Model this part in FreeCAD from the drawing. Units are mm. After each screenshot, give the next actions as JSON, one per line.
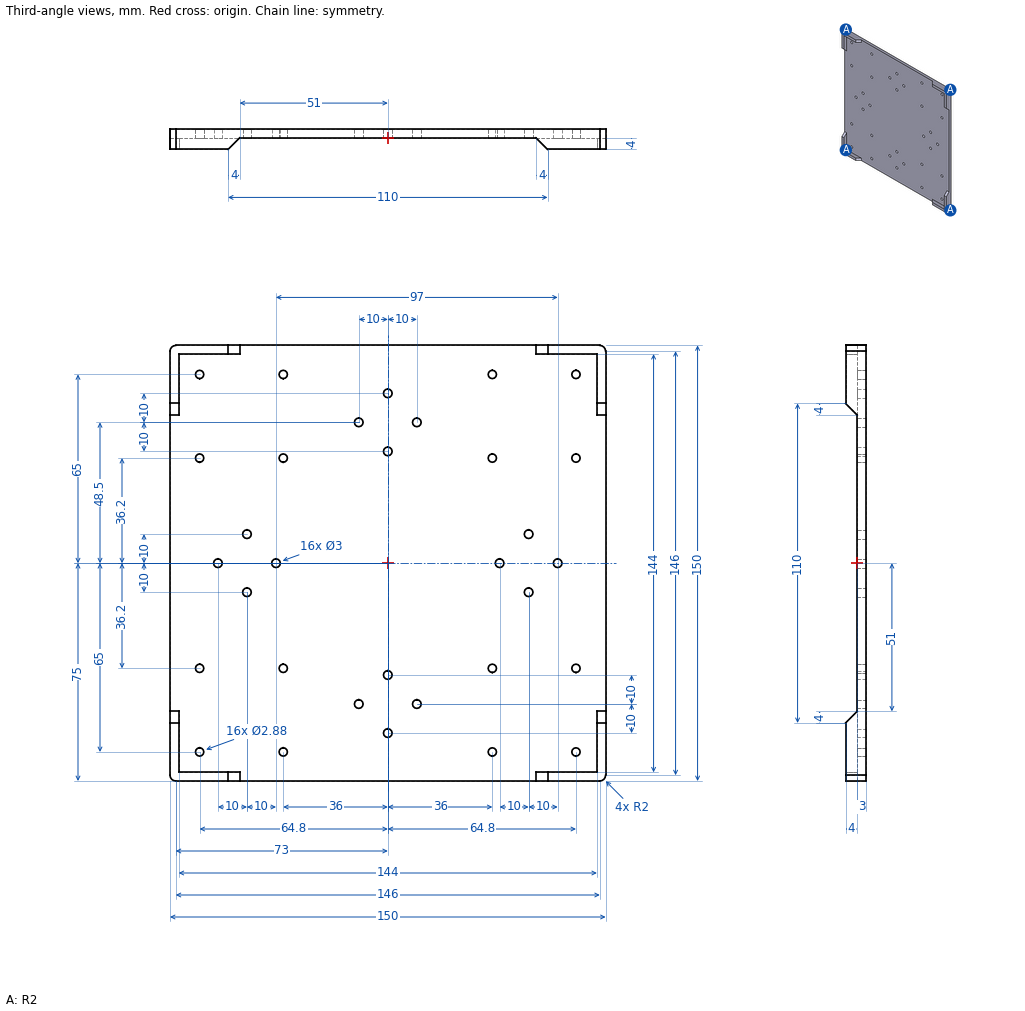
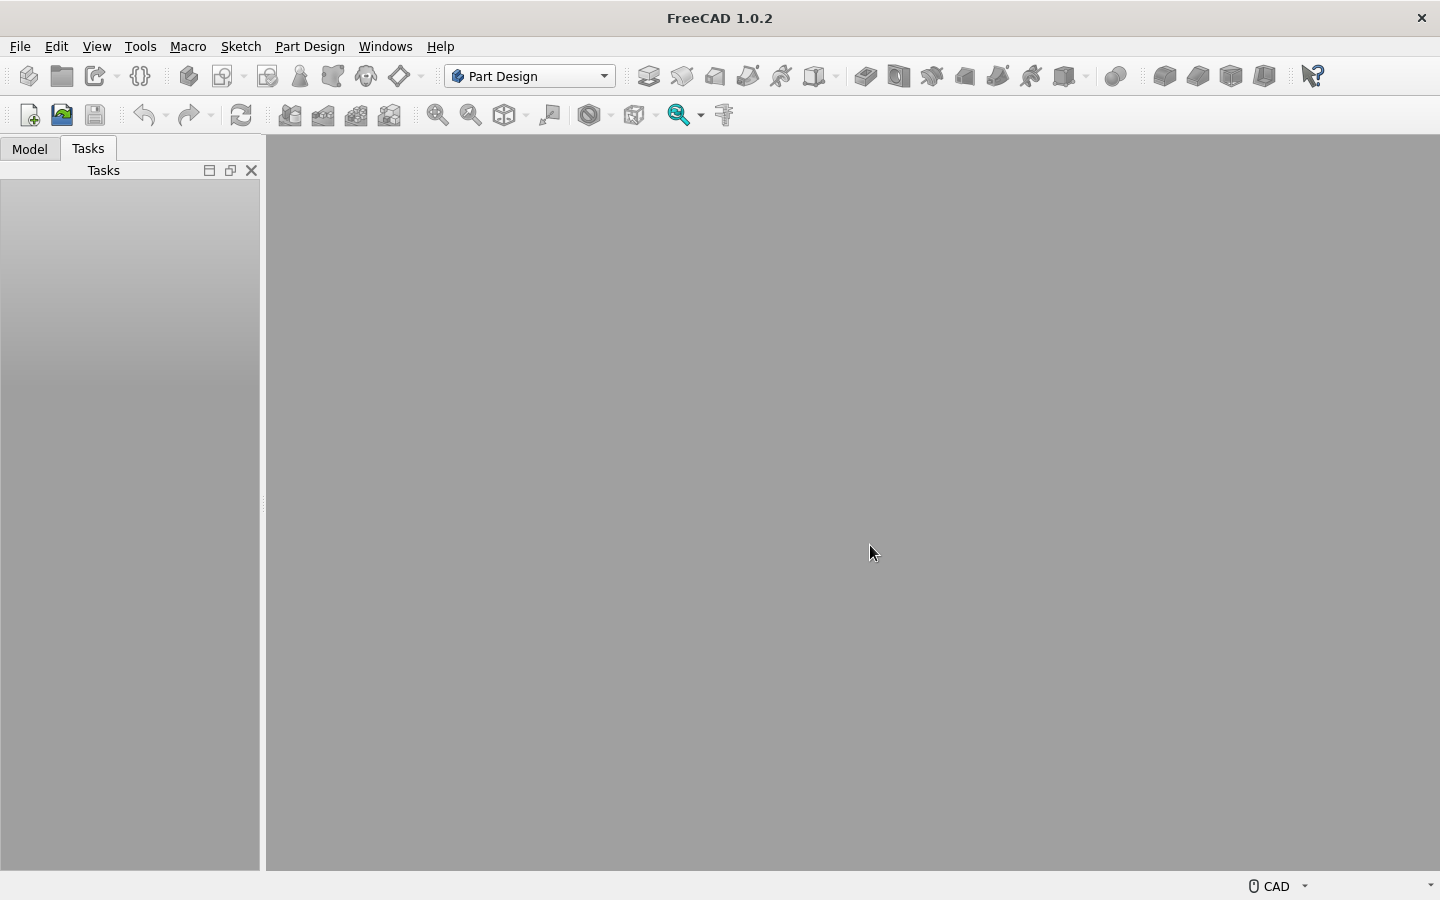
{"action": "left_click", "coordinate": [29, 116]}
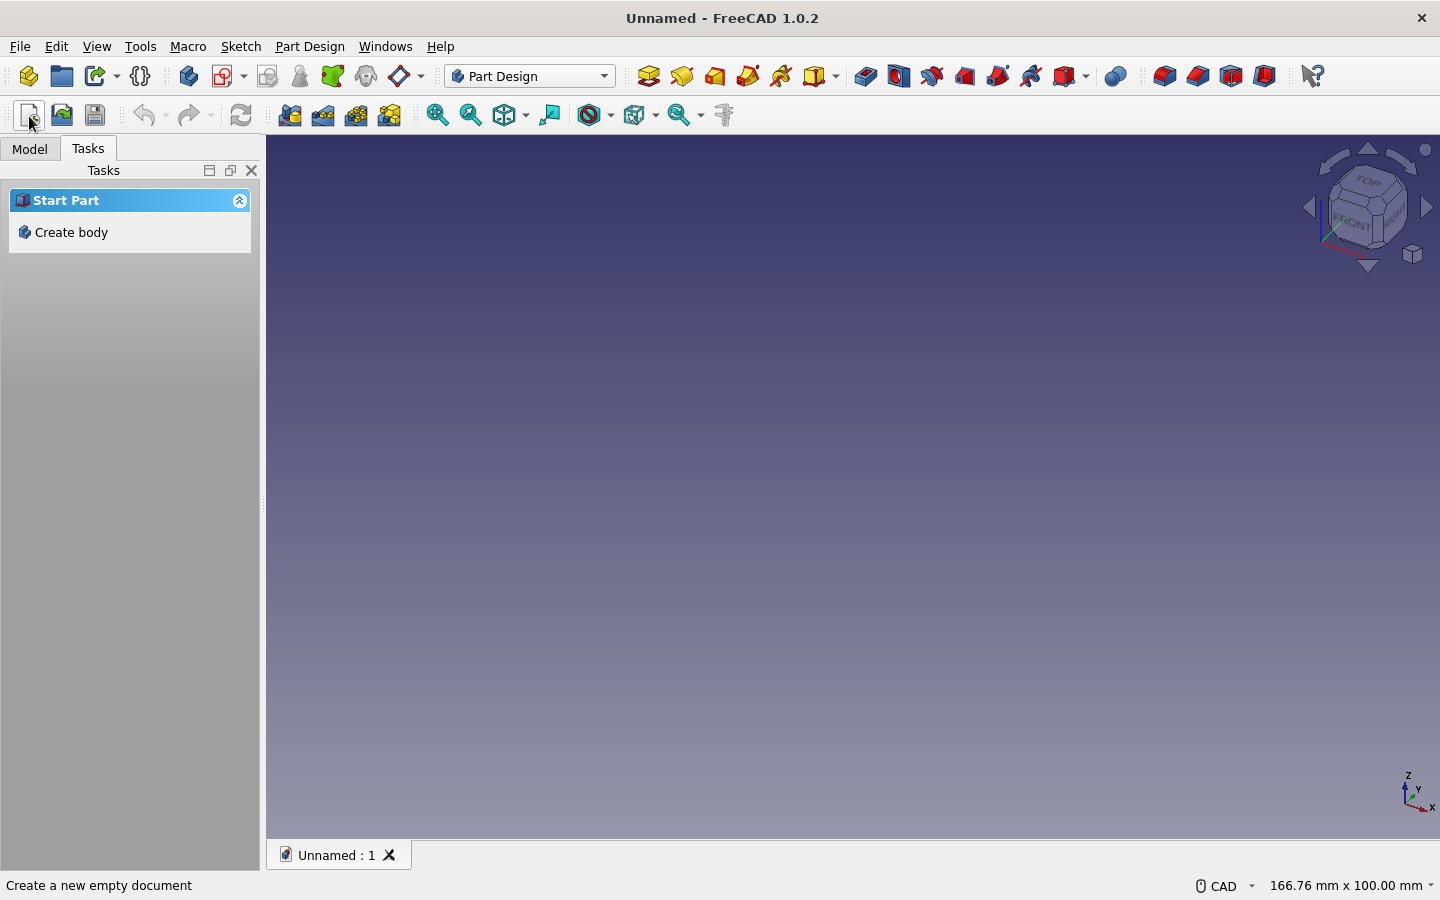
{"action": "left_click", "coordinate": [222, 76]}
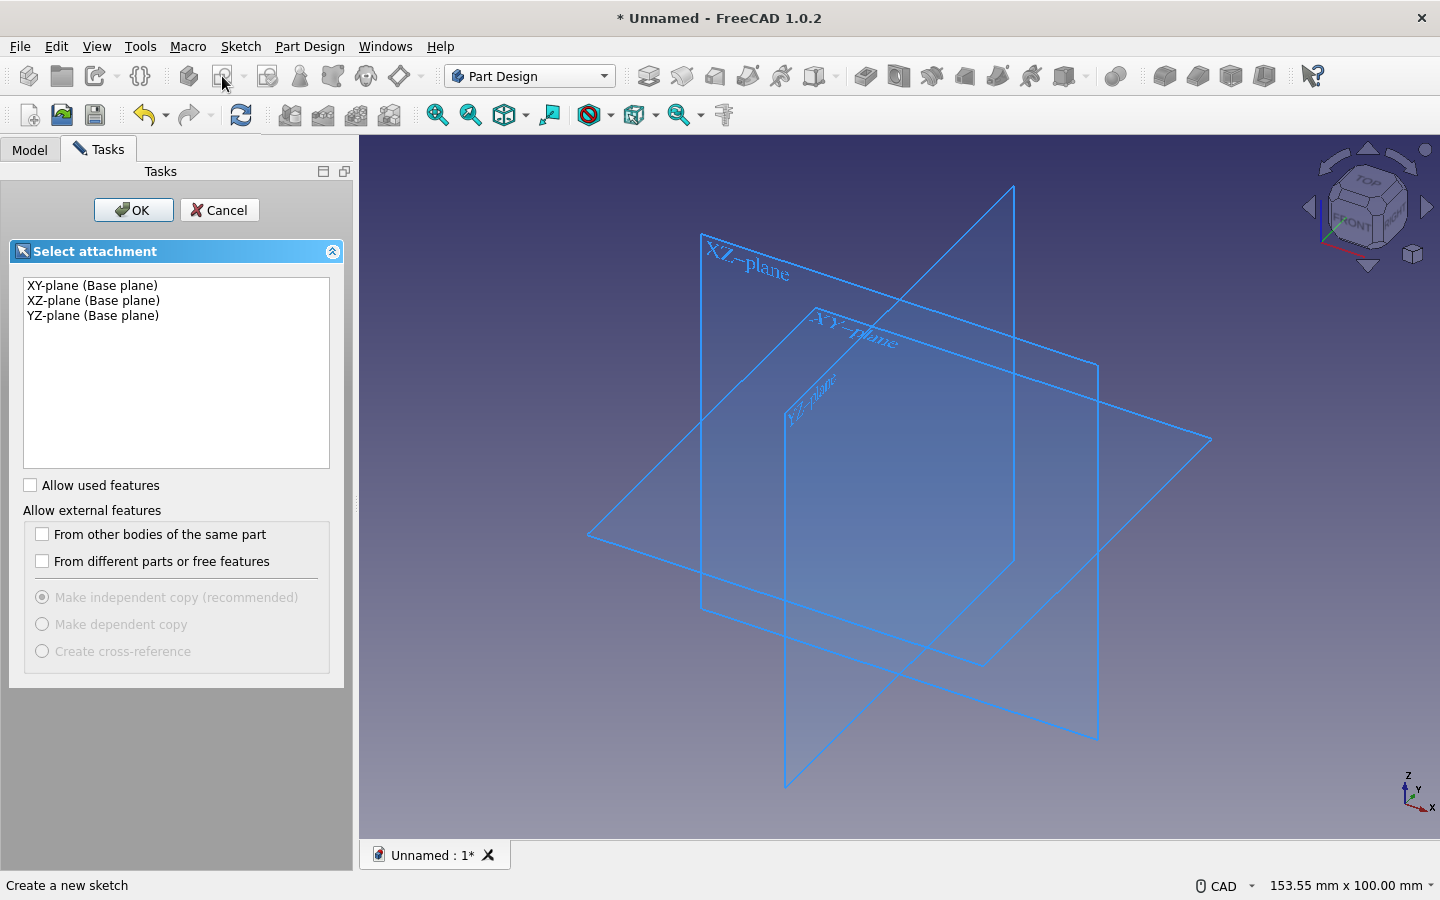
{"action": "left_click", "coordinate": [84, 300]}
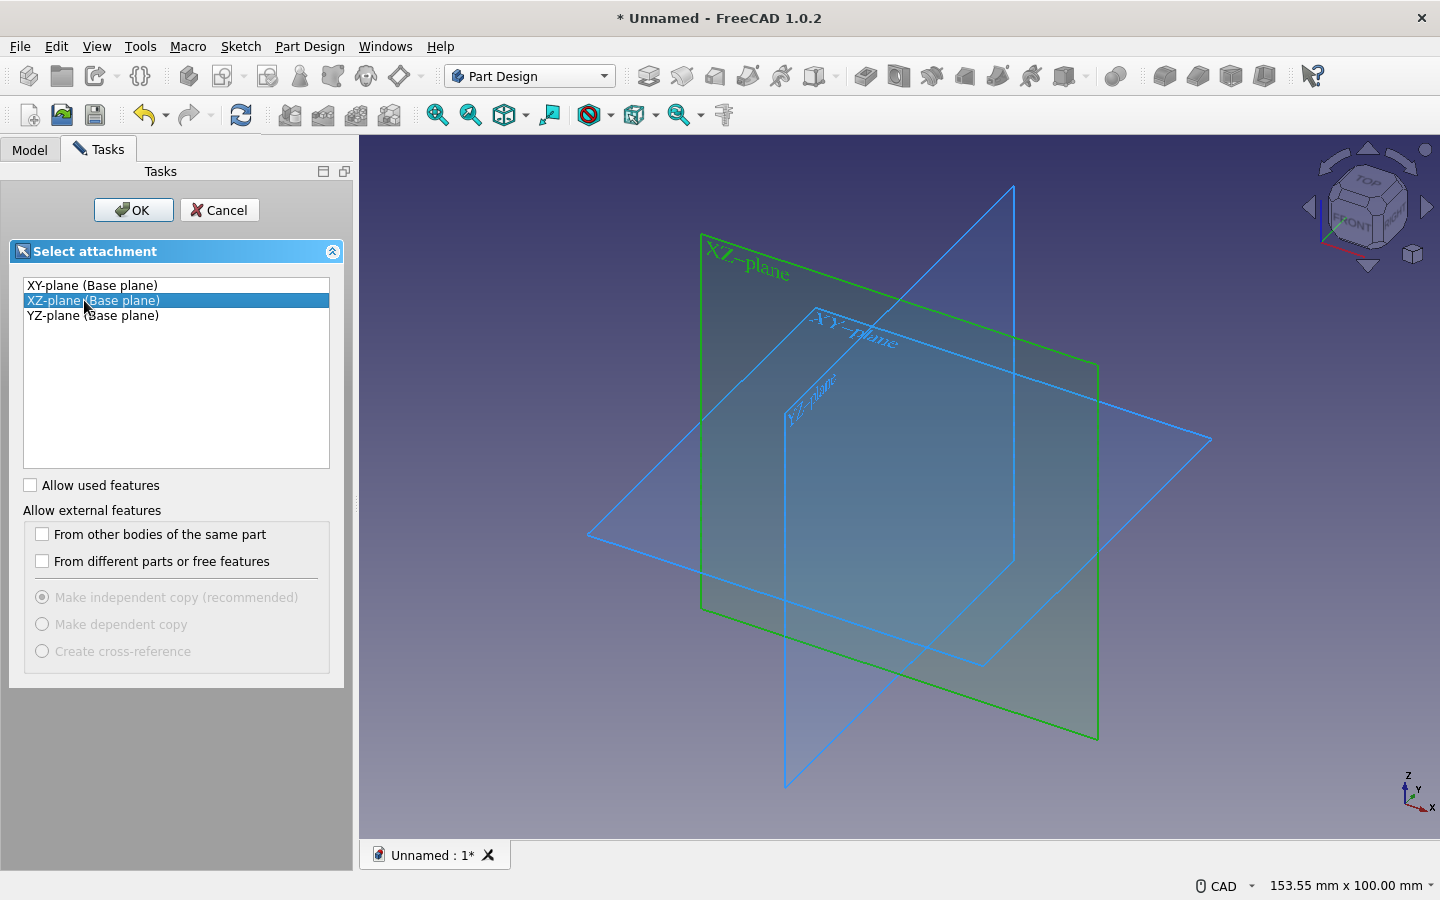
{"action": "left_click", "coordinate": [134, 210]}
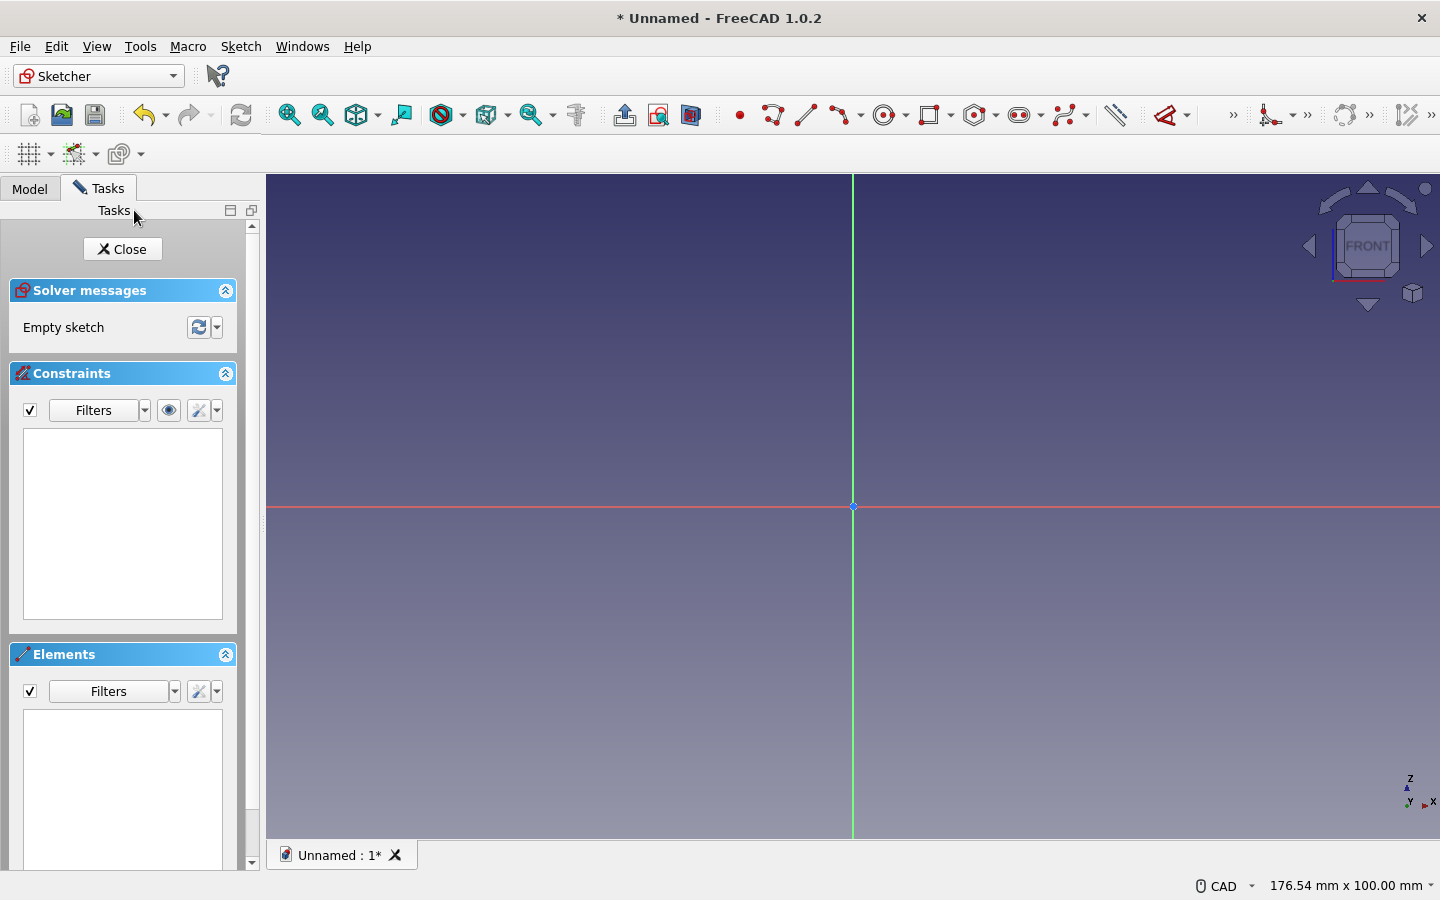
{"action": "scroll", "coordinate": [729, 506], "scroll_direction": "down", "scroll_amount": 4}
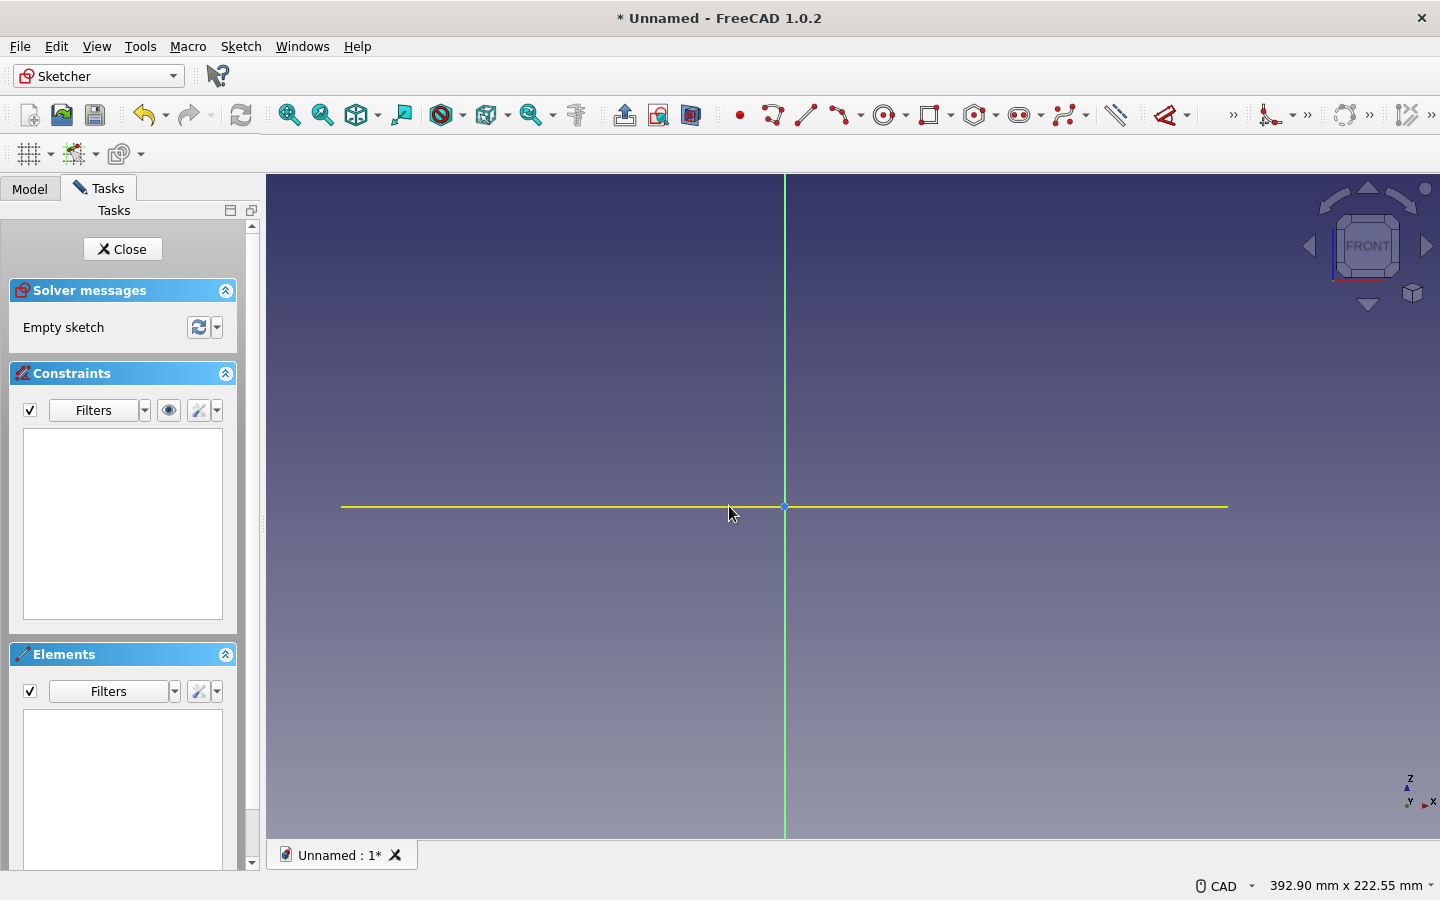
{"action": "key", "text": "g v"}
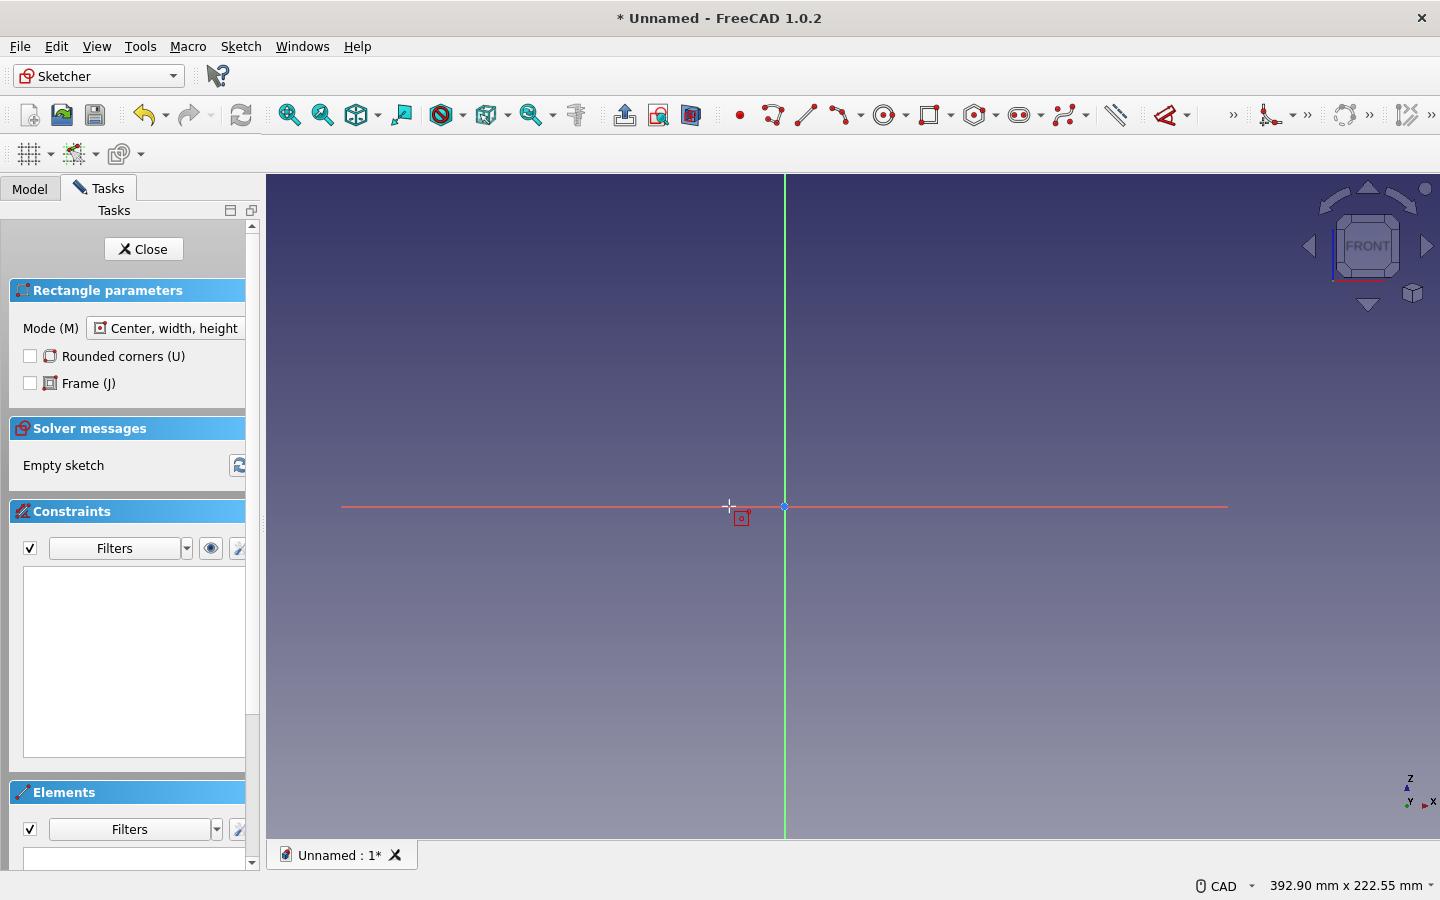
{"action": "left_click", "coordinate": [785, 506]}
{"action": "left_click", "coordinate": [1009, 282]}
{"action": "key", "text": "Escape"}